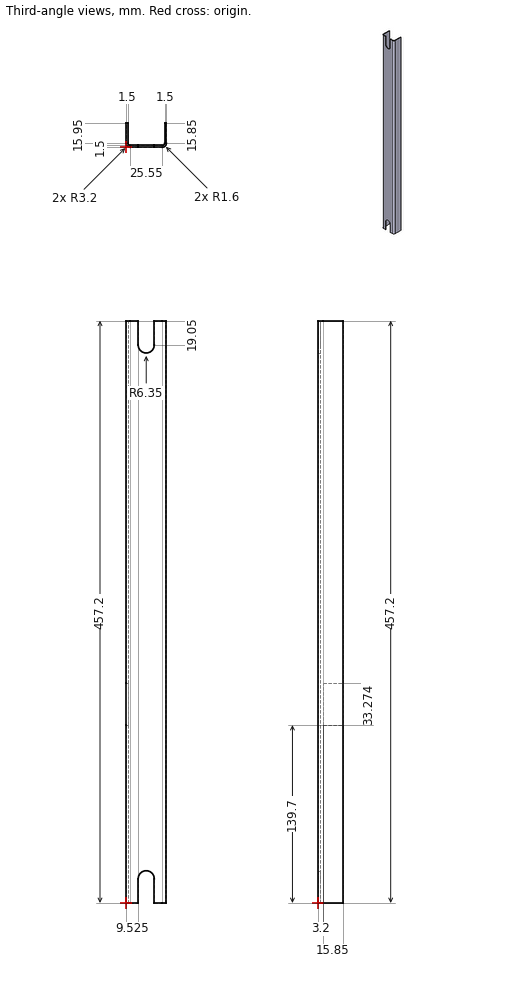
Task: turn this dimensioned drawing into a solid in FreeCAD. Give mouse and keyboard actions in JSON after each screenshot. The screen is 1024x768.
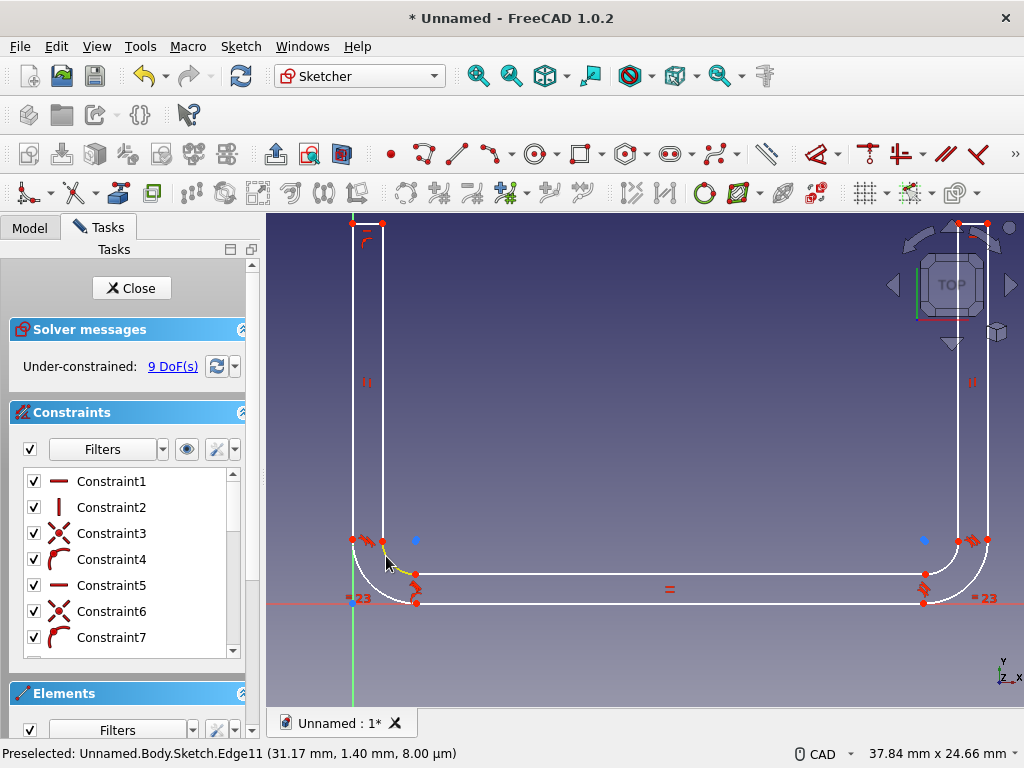
{"action": "left_click", "coordinate": [386, 556]}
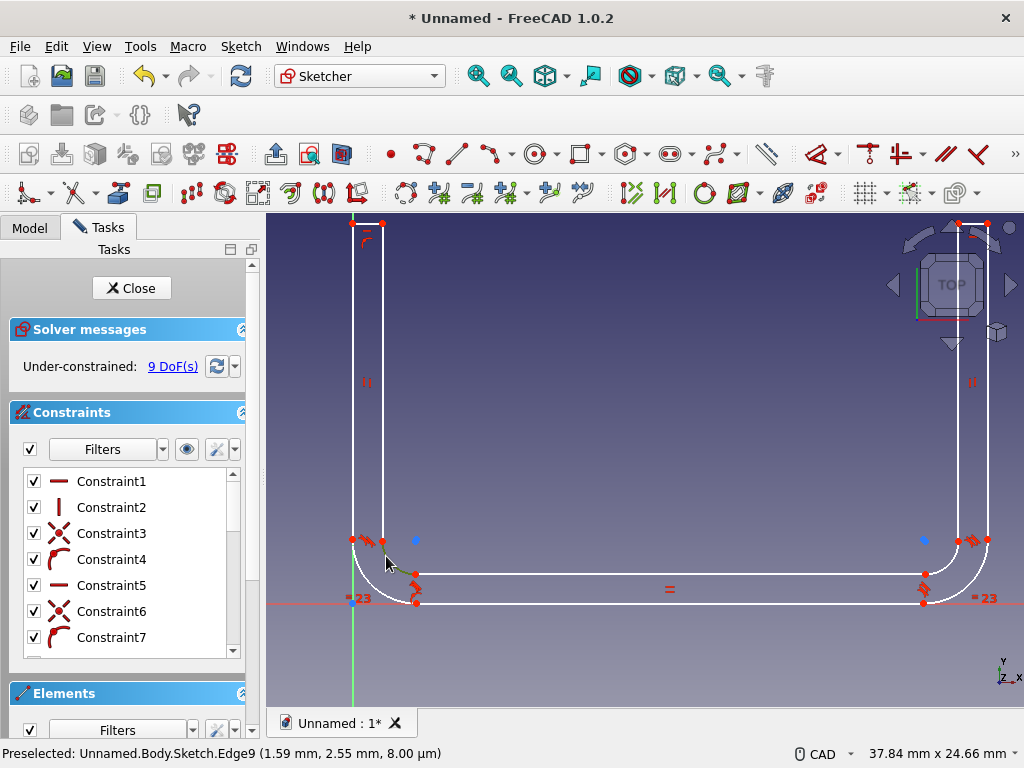
{"action": "scroll", "coordinate": [385, 556], "scroll_direction": "down", "scroll_amount": 2}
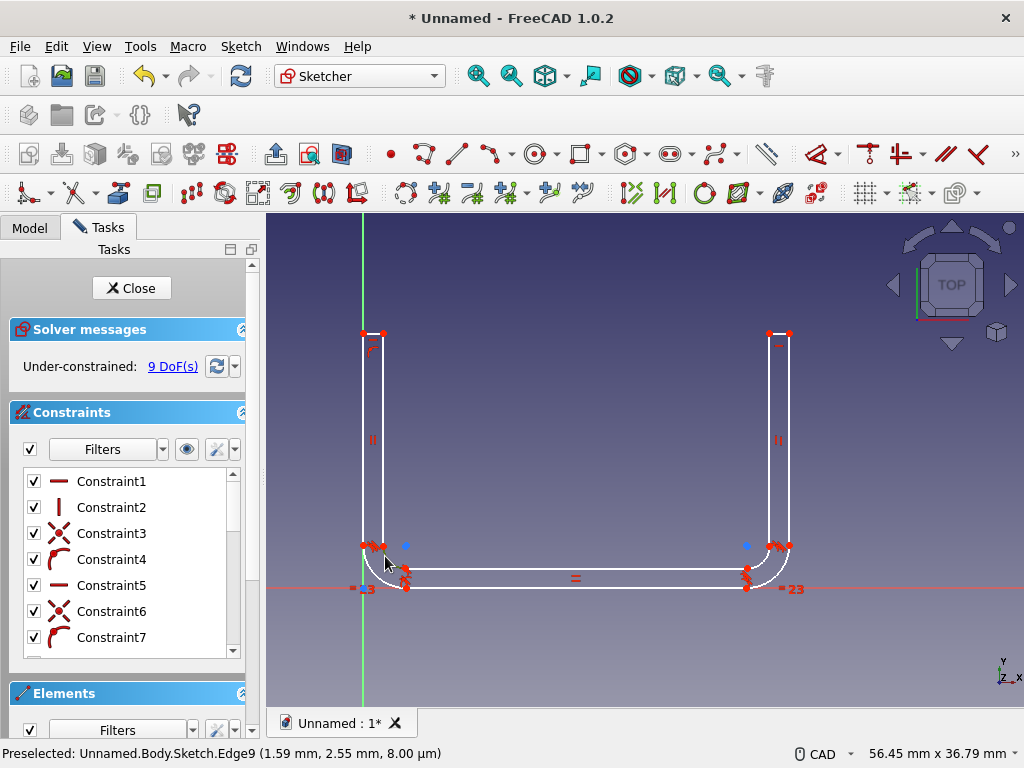
{"action": "scroll", "coordinate": [757, 566], "scroll_direction": "up", "scroll_amount": 2}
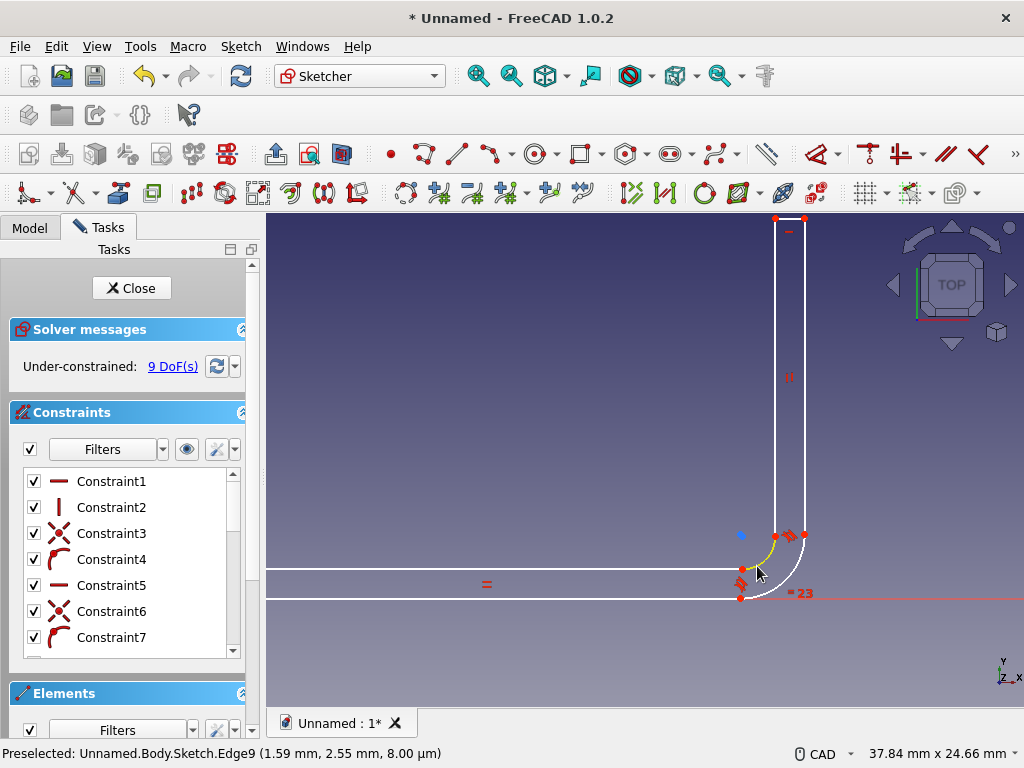
{"action": "left_click", "coordinate": [757, 566]}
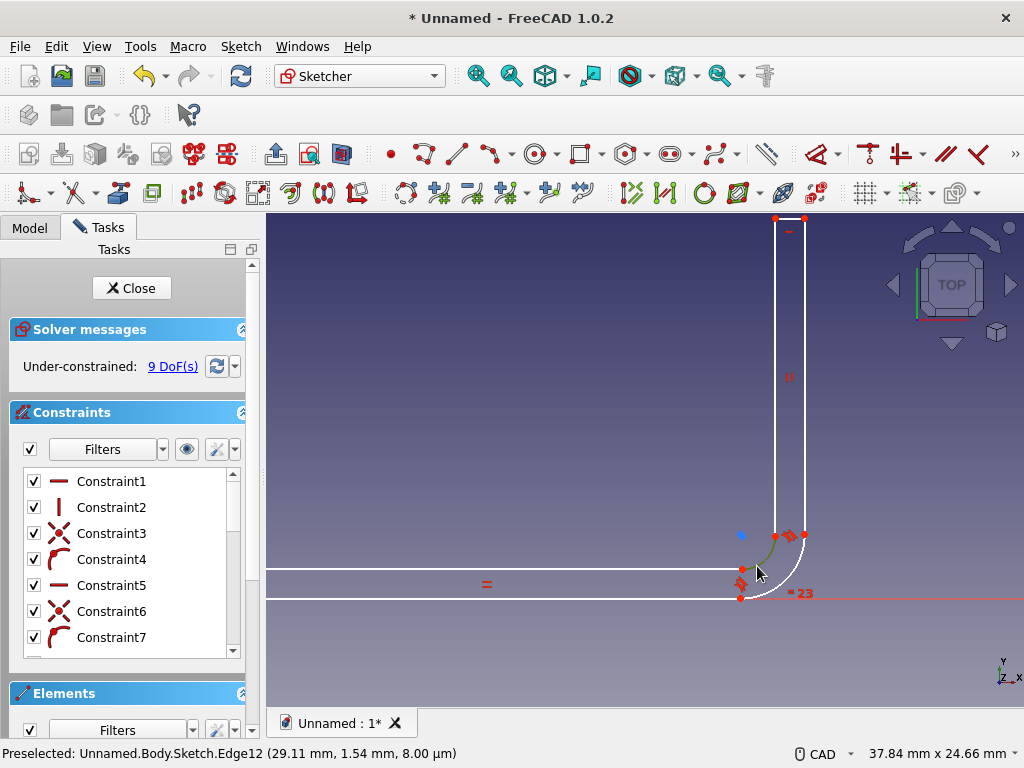
{"action": "key", "text": "e"}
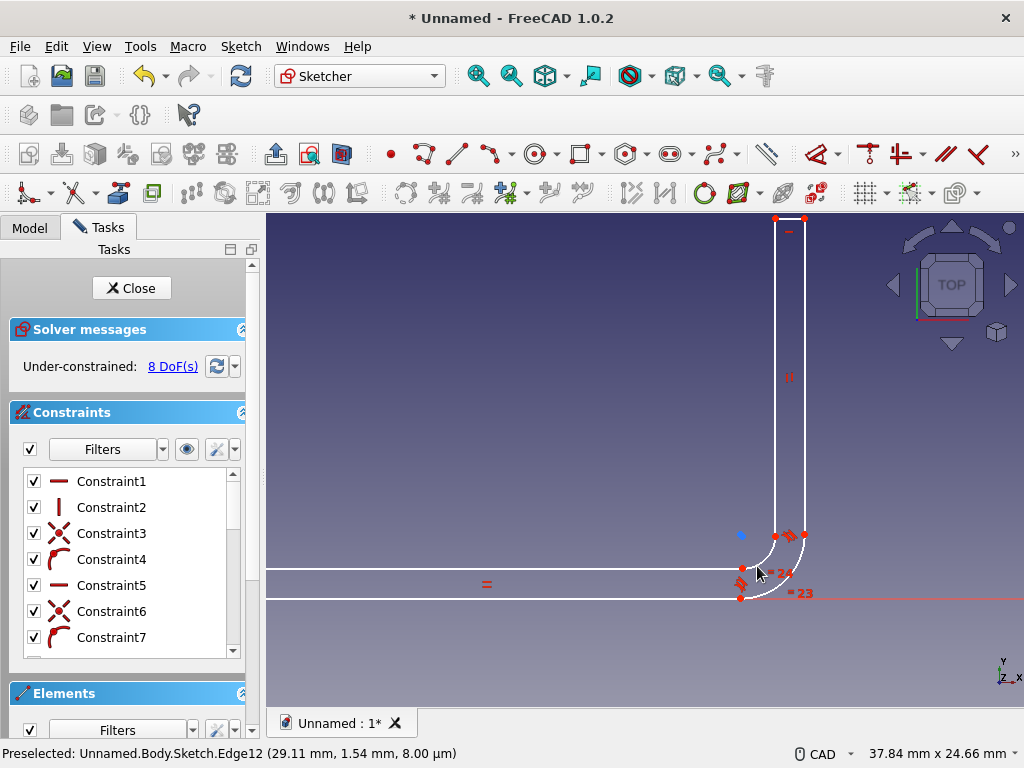
{"action": "key", "text": "d"}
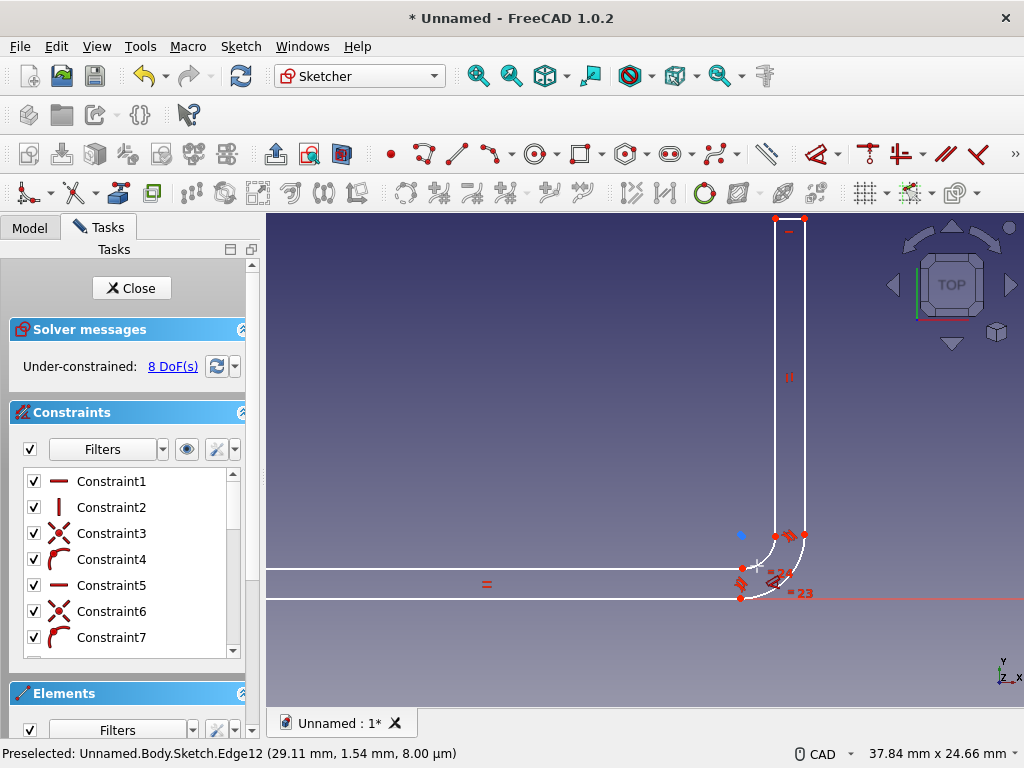
{"action": "scroll", "coordinate": [758, 566], "scroll_direction": "down", "scroll_amount": 2}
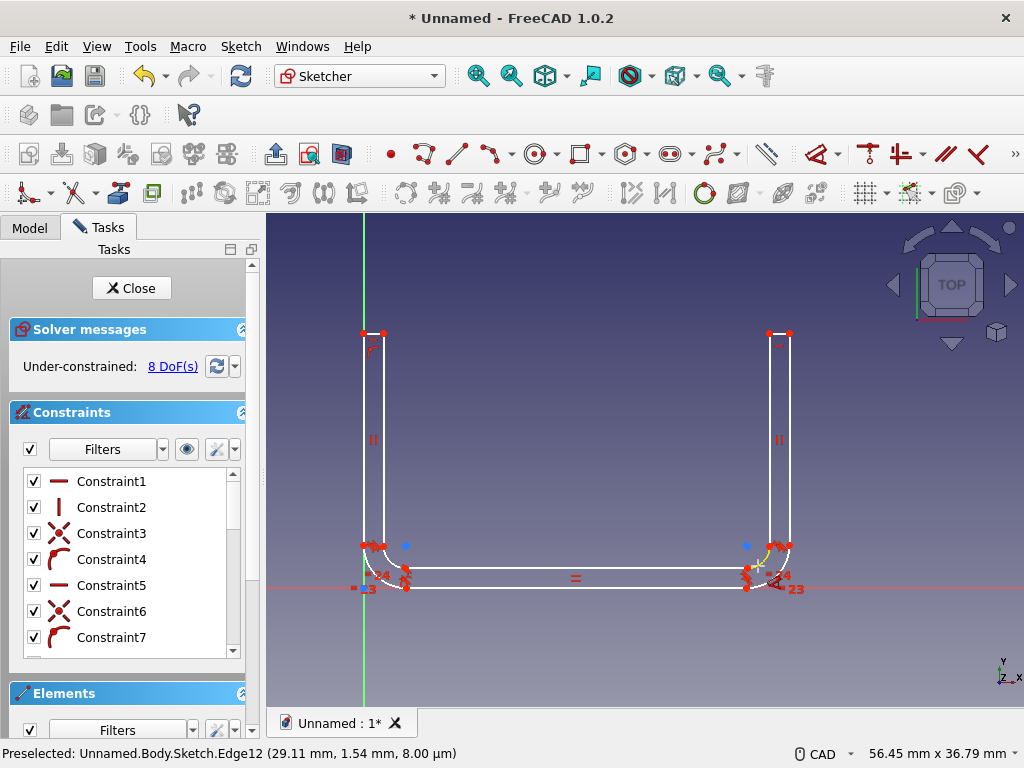
{"action": "scroll", "coordinate": [386, 556], "scroll_direction": "up", "scroll_amount": 4}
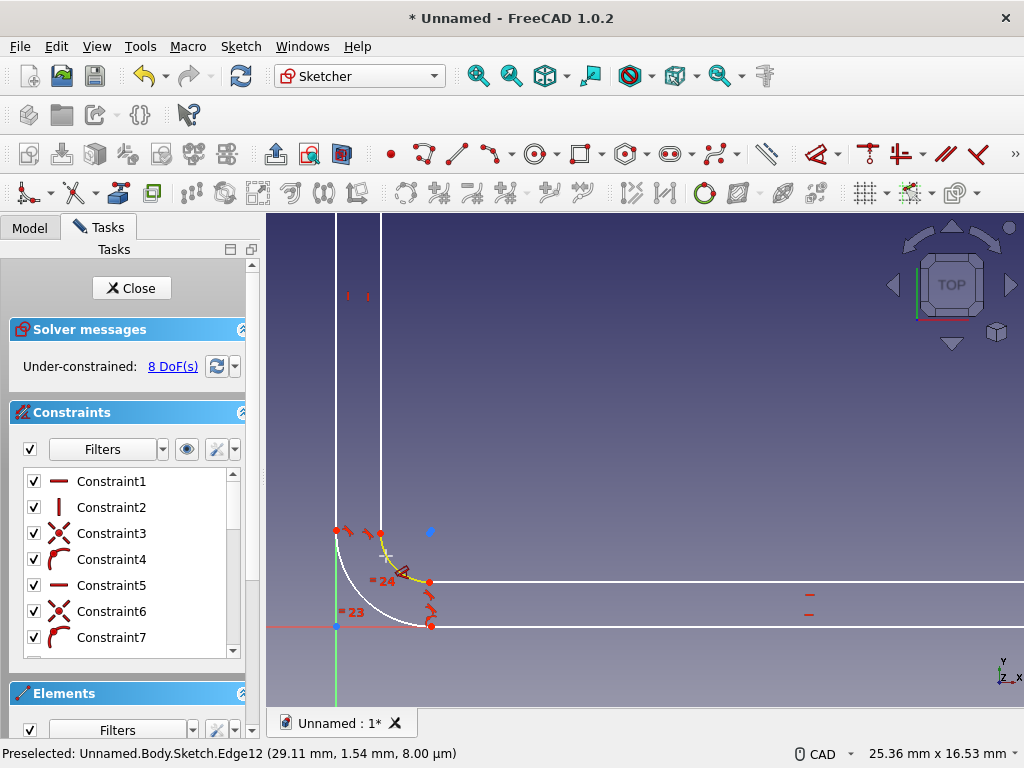
{"action": "left_click", "coordinate": [386, 556]}
{"action": "left_click", "coordinate": [359, 493]}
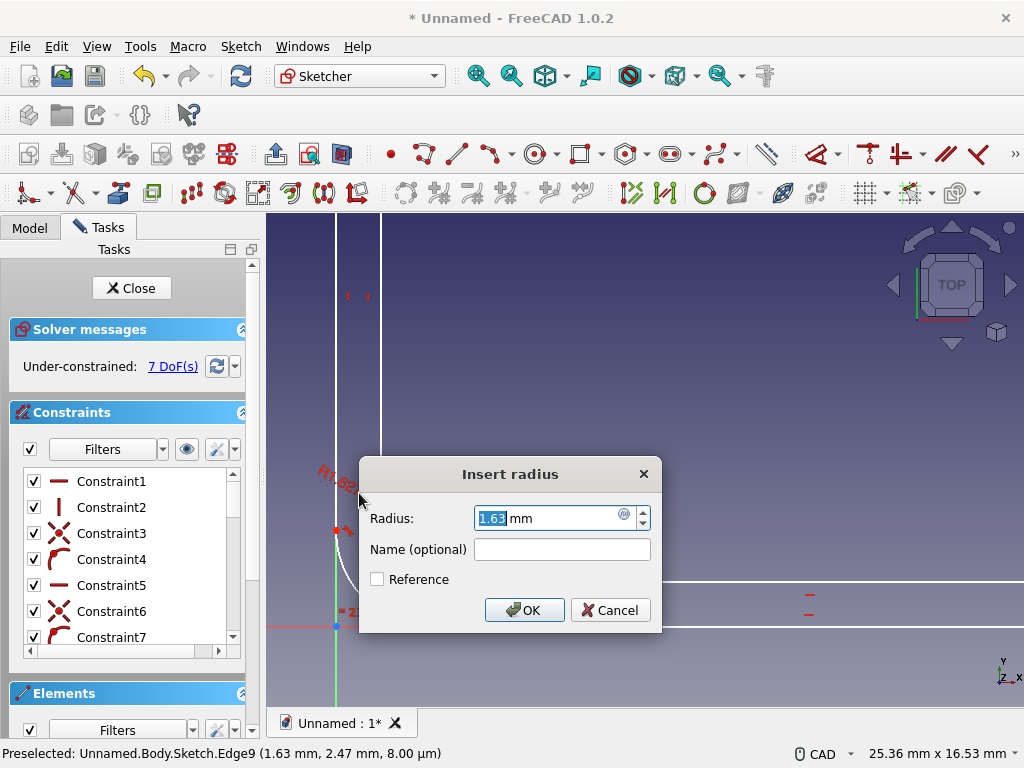
{"action": "type", "text": "1.6"}
{"action": "key", "text": "Return"}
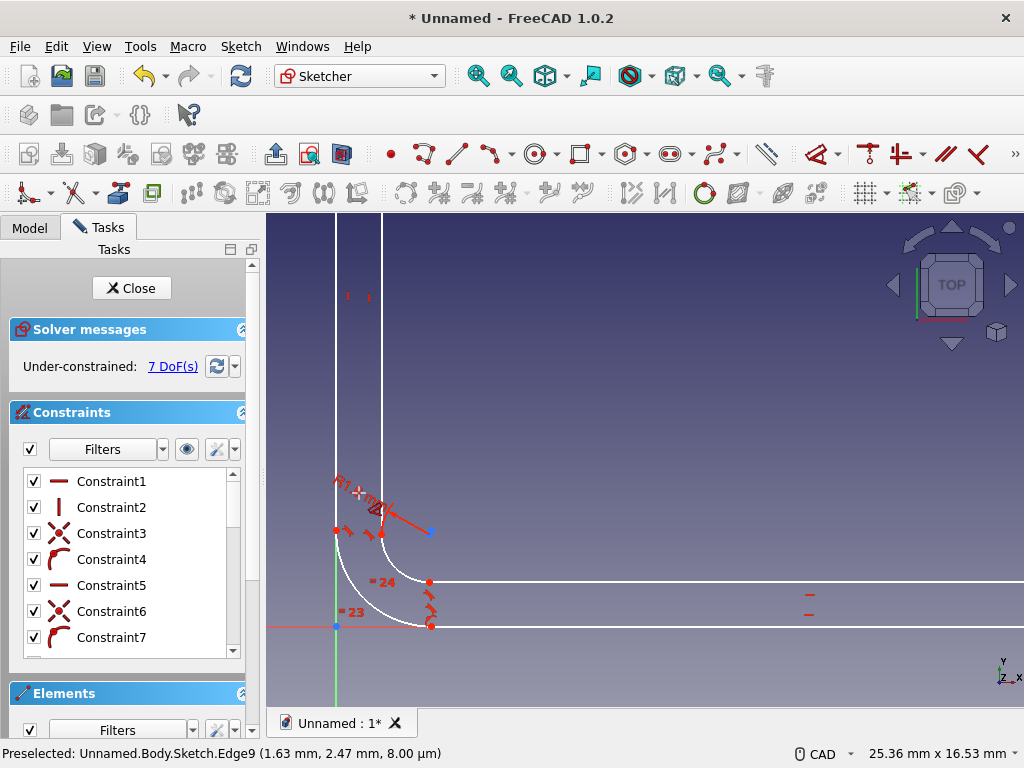
{"action": "scroll", "coordinate": [347, 574], "scroll_direction": "up", "scroll_amount": 2}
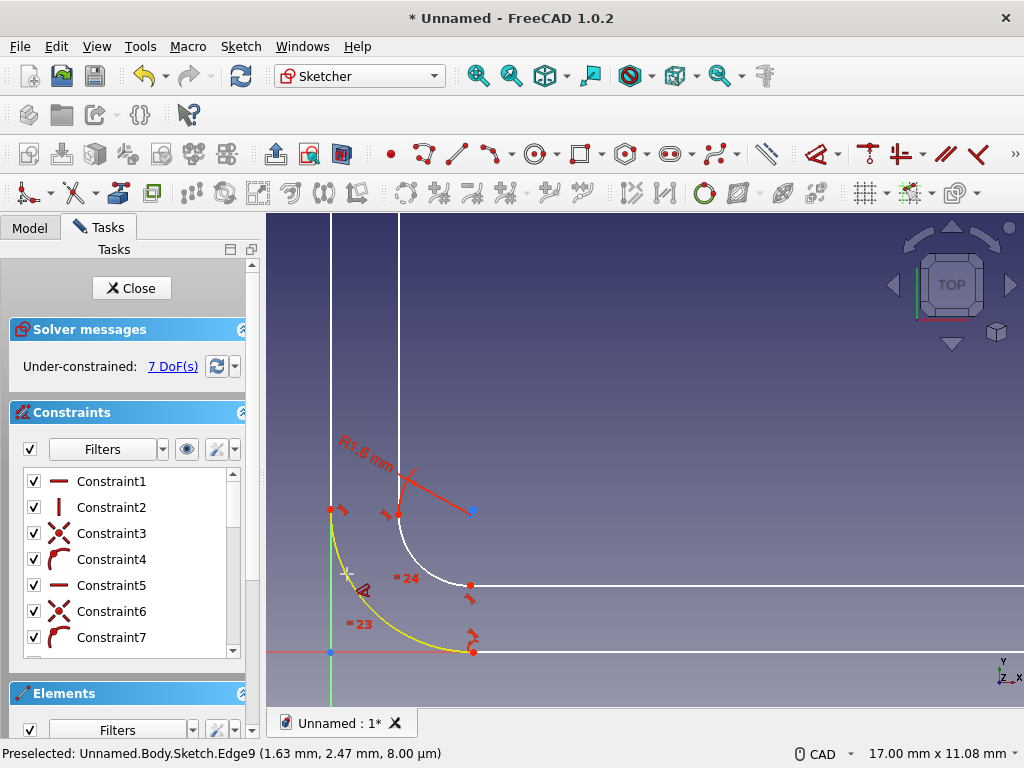
{"action": "left_click", "coordinate": [346, 574]}
{"action": "left_click", "coordinate": [317, 588]}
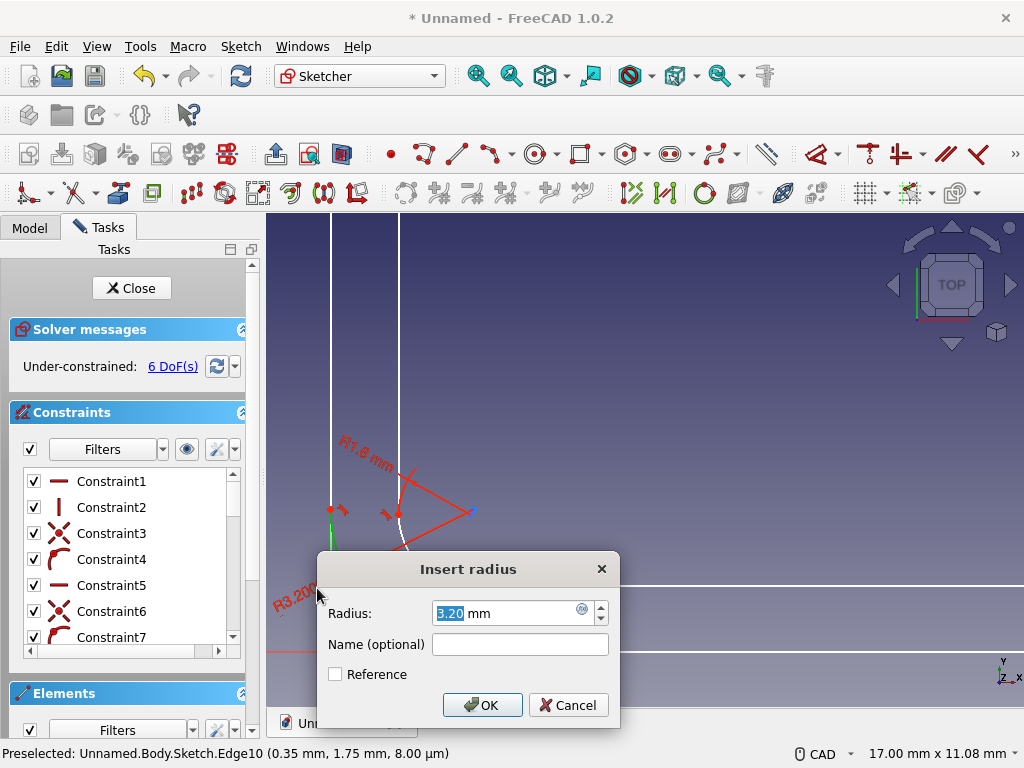
{"action": "type", "text": "3.2"}
{"action": "key", "text": "Return"}